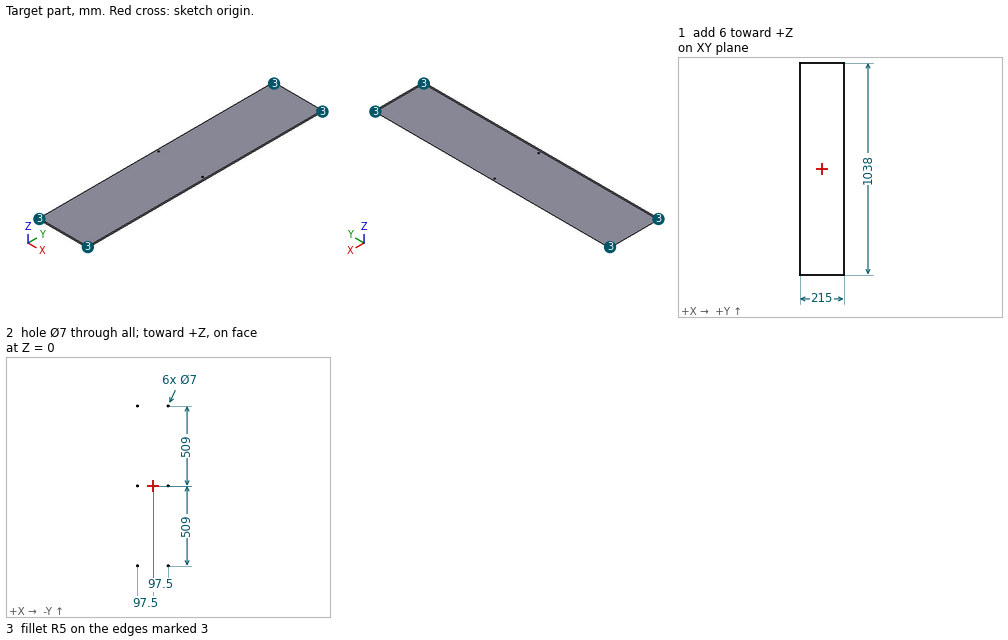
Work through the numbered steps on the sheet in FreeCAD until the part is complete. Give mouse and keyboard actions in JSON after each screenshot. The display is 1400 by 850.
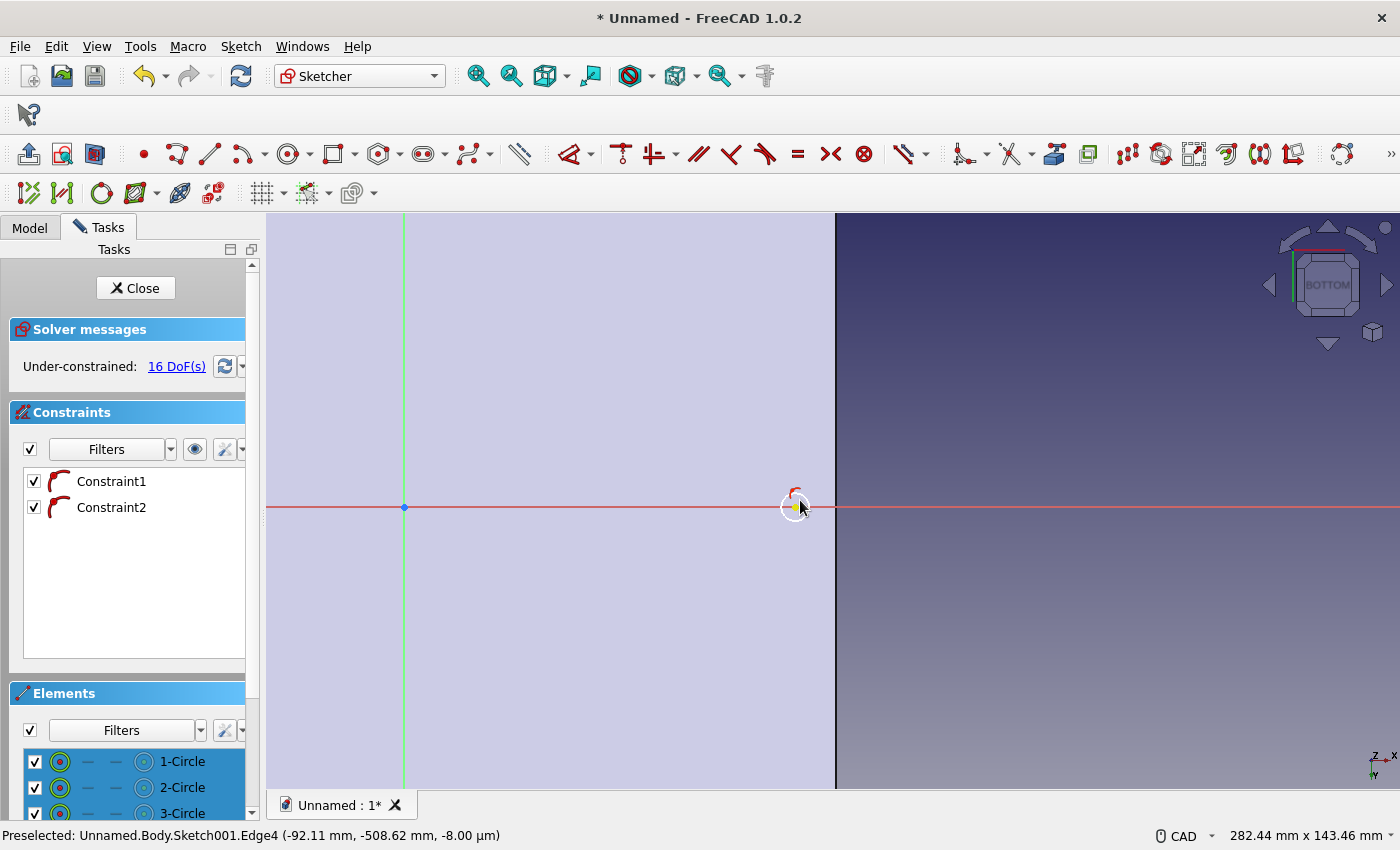
{"action": "left_click", "coordinate": [781, 507]}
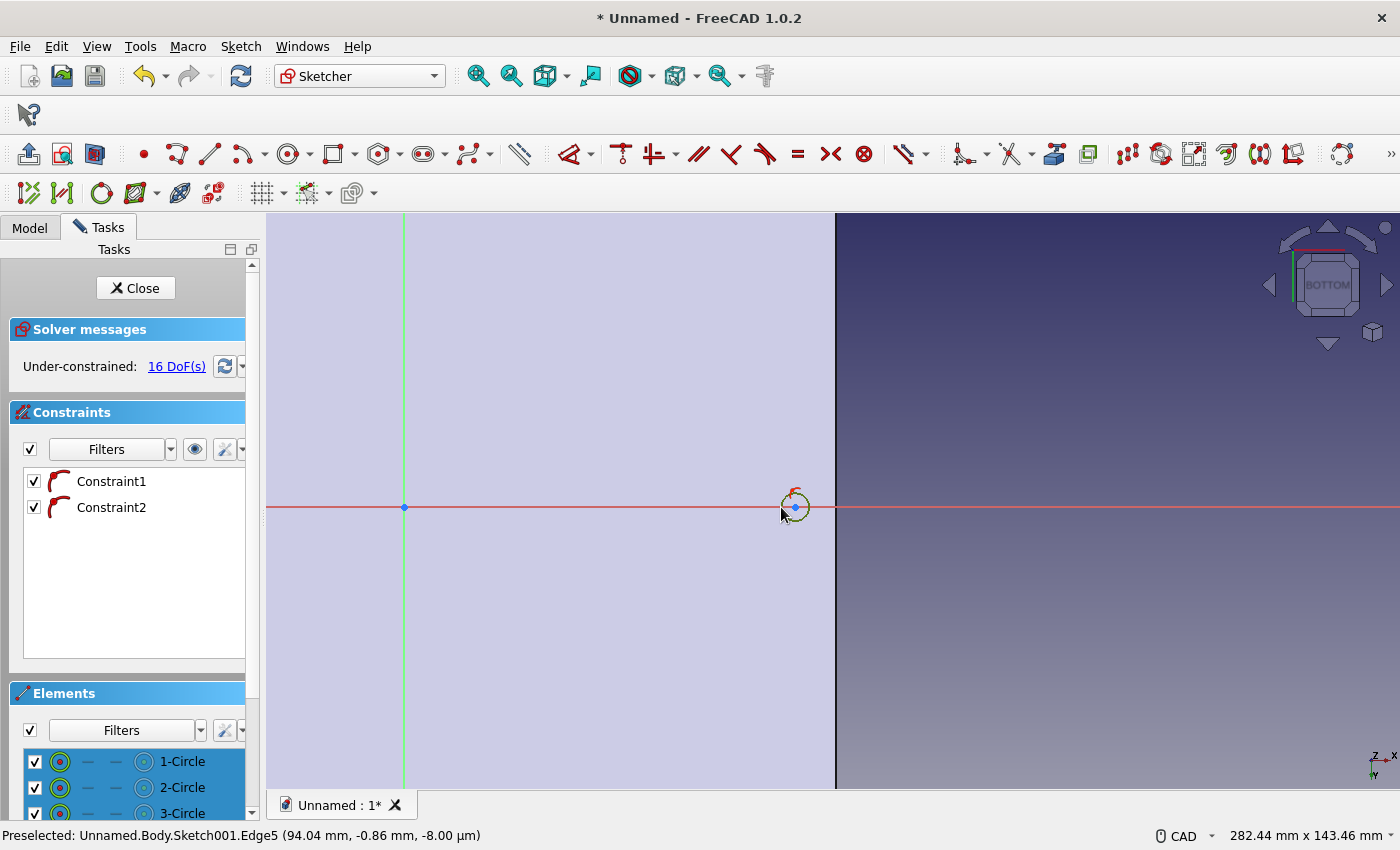
{"action": "scroll", "coordinate": [800, 500], "scroll_direction": "down", "scroll_amount": 12}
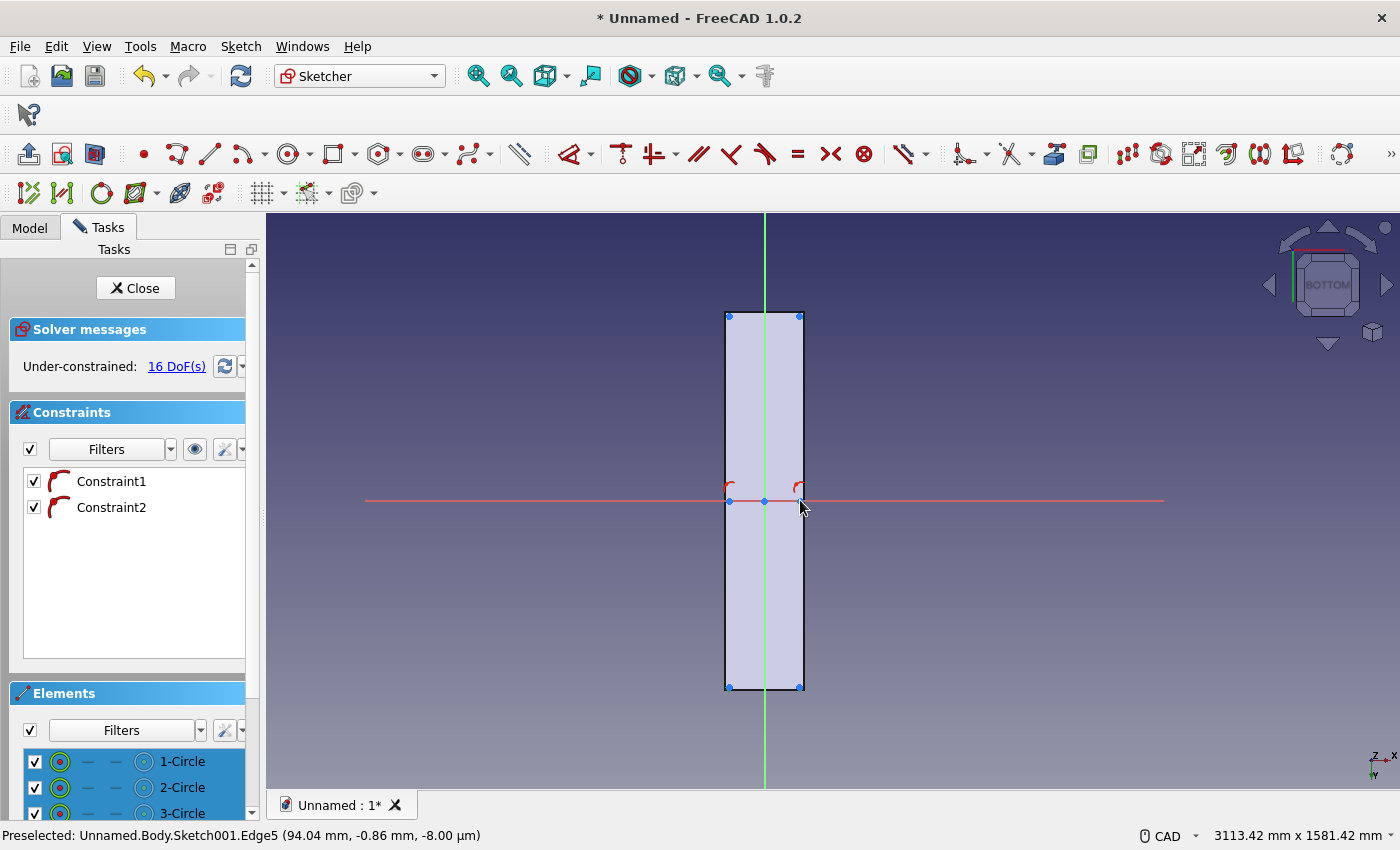
{"action": "scroll", "coordinate": [730, 500], "scroll_direction": "up", "scroll_amount": 14}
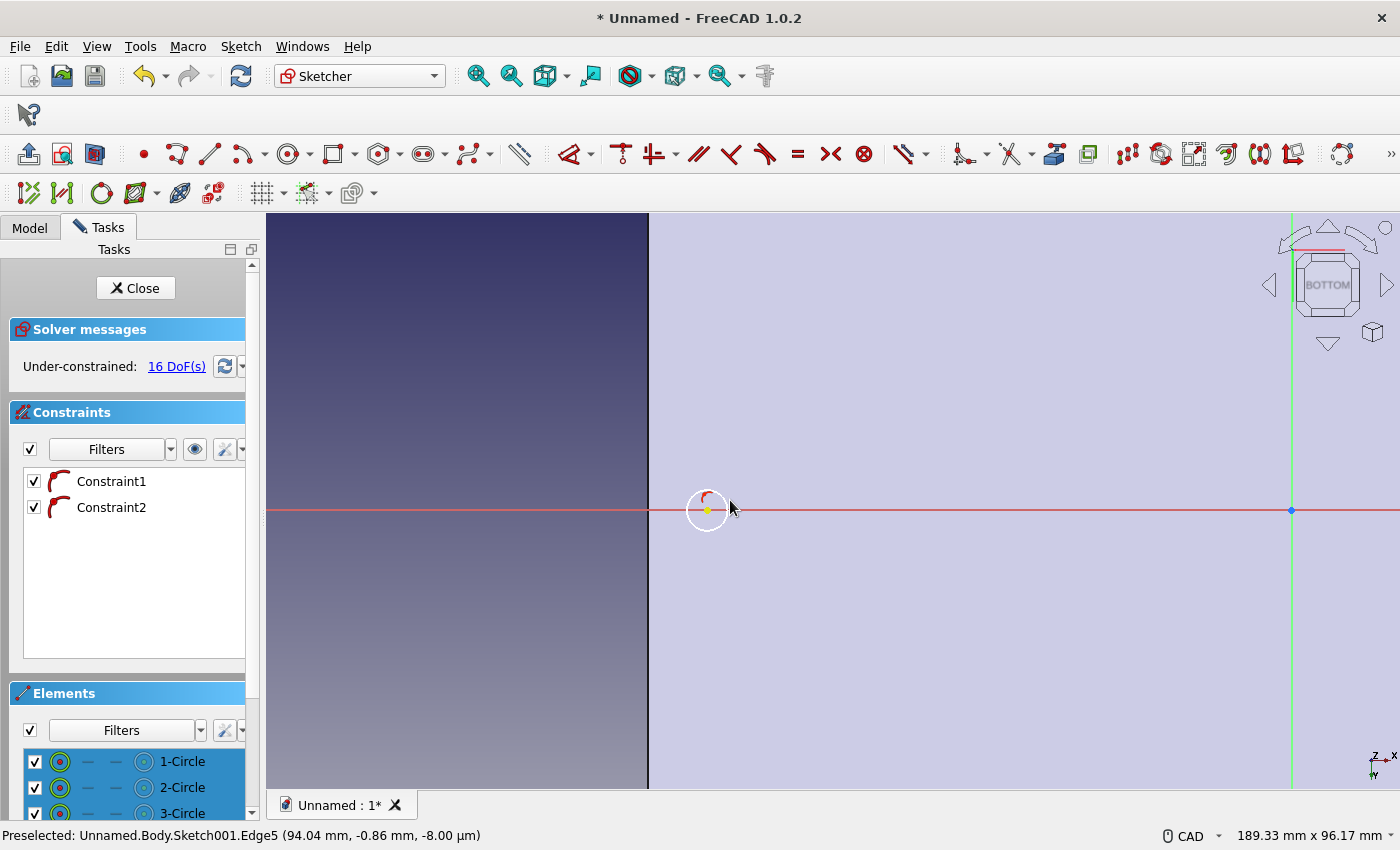
{"action": "left_click", "coordinate": [722, 496]}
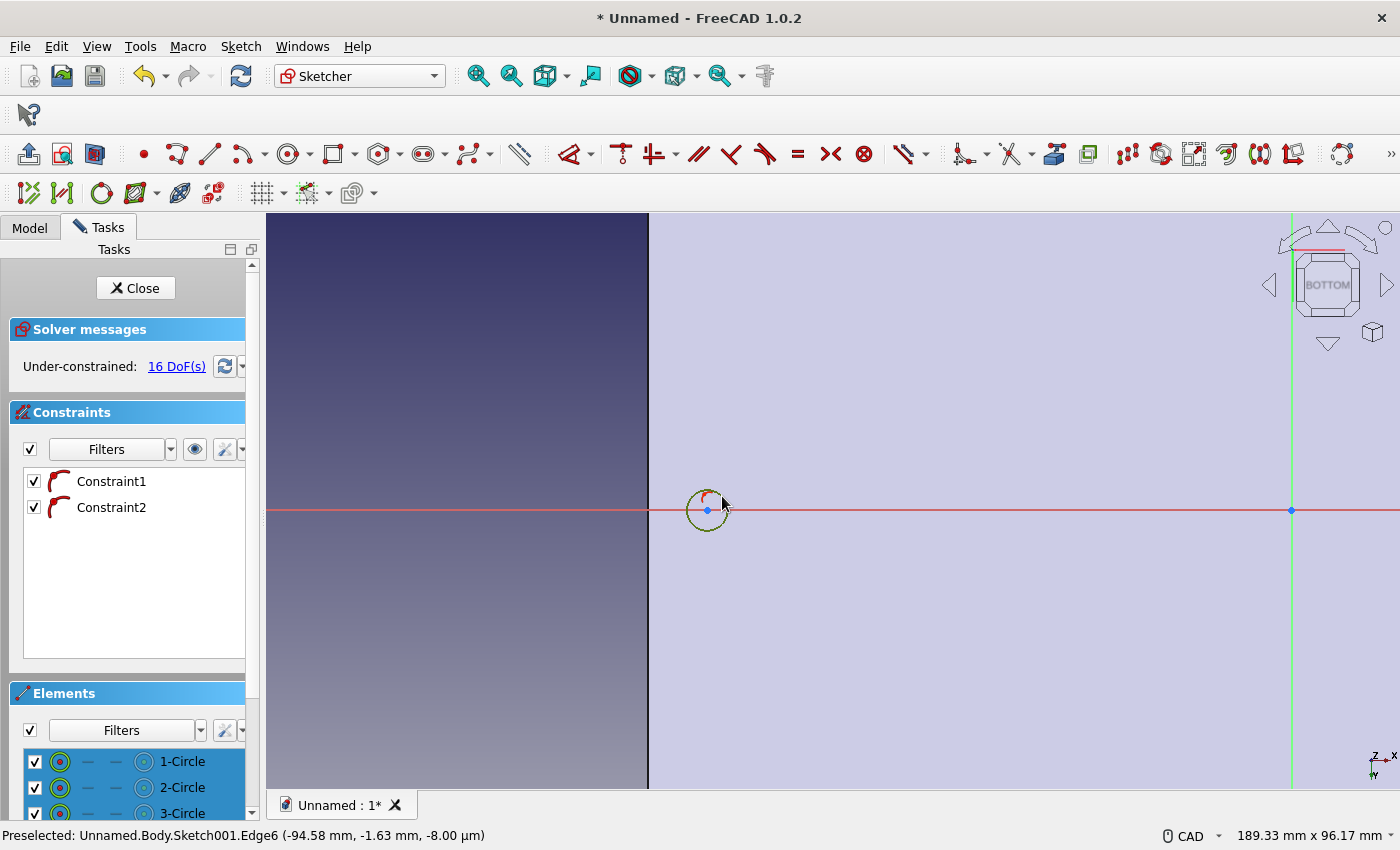
{"action": "left_click", "coordinate": [798, 154]}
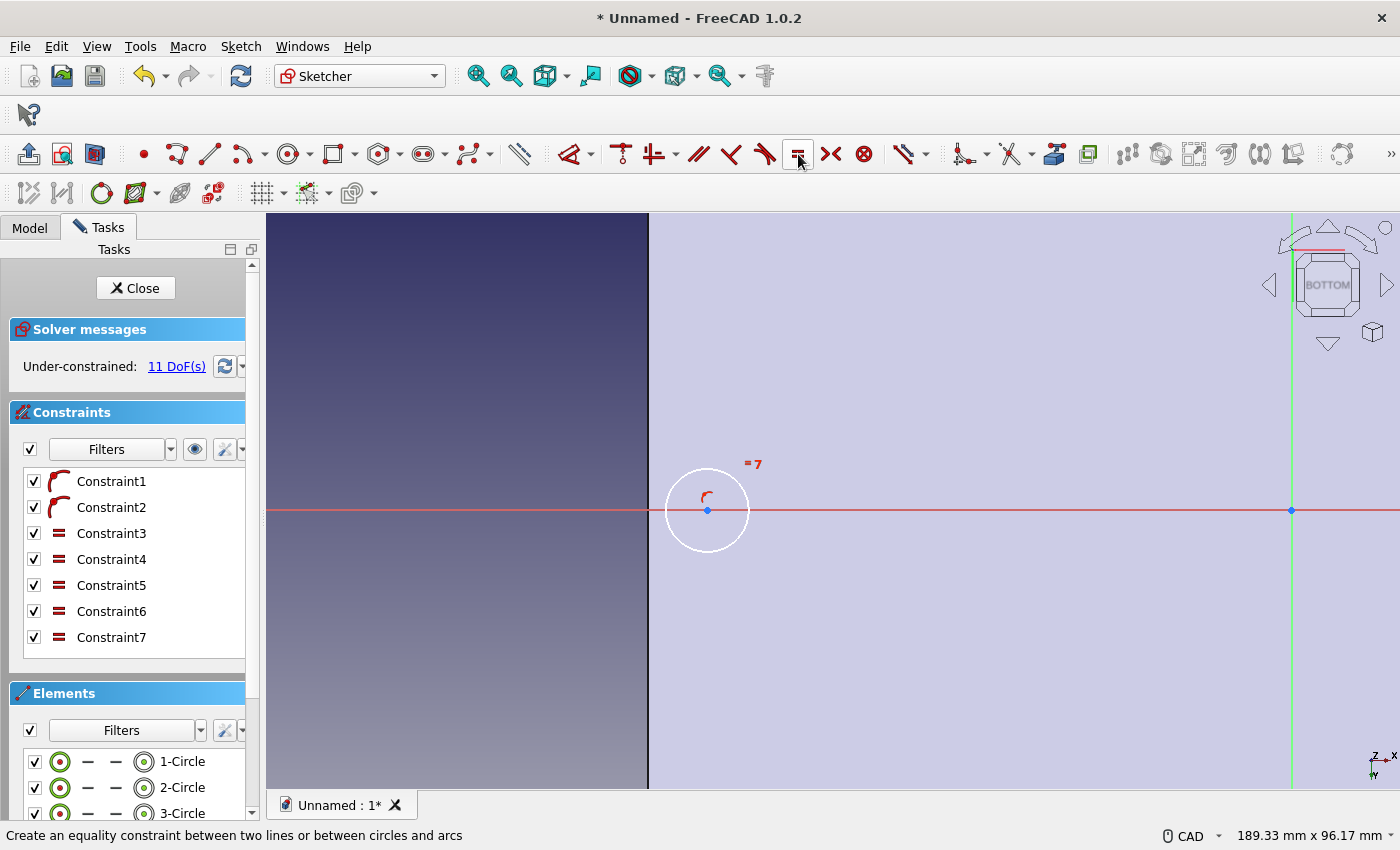
{"action": "scroll", "coordinate": [730, 500], "scroll_direction": "down", "scroll_amount": 14}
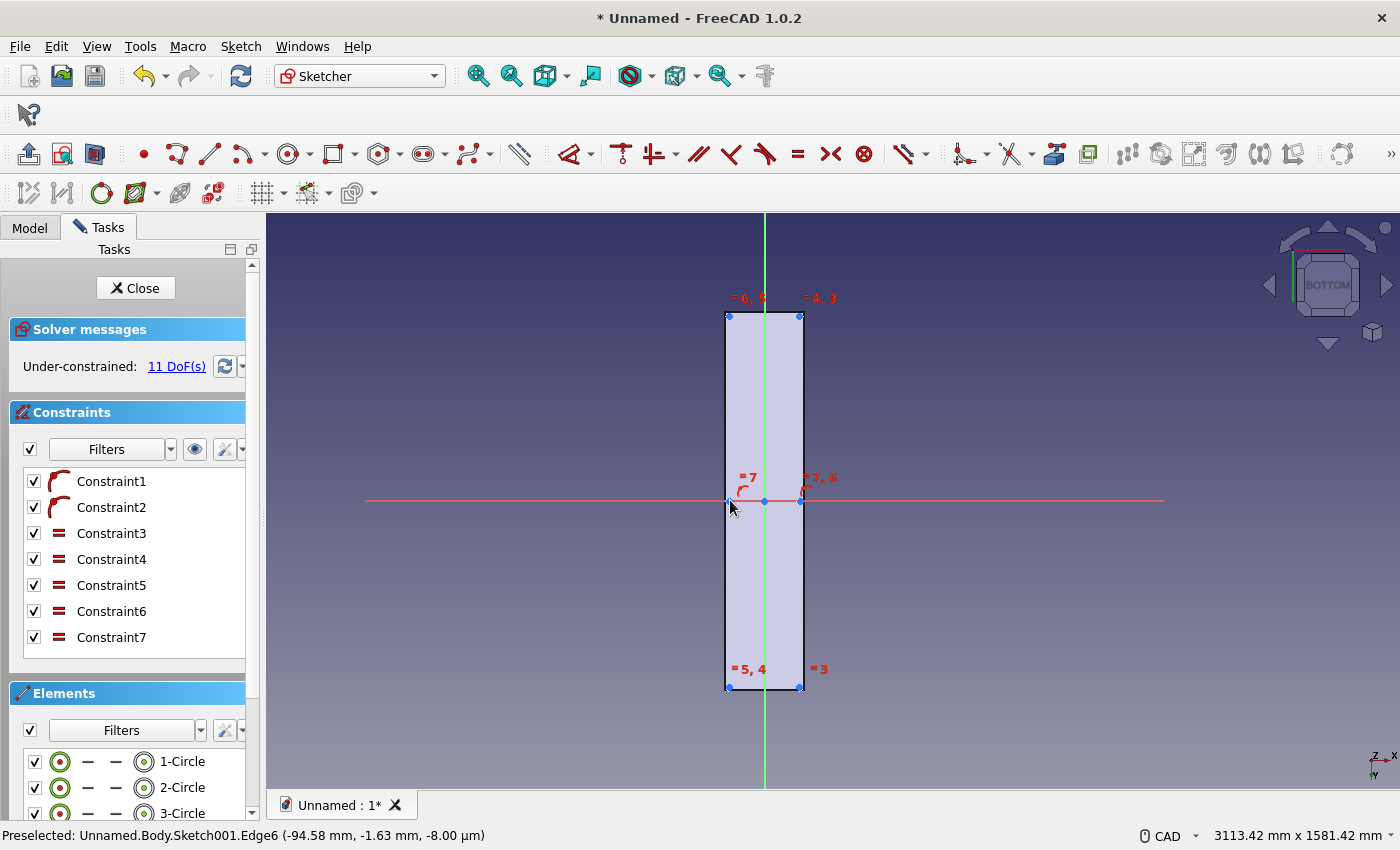
{"action": "left_click", "coordinate": [800, 688]}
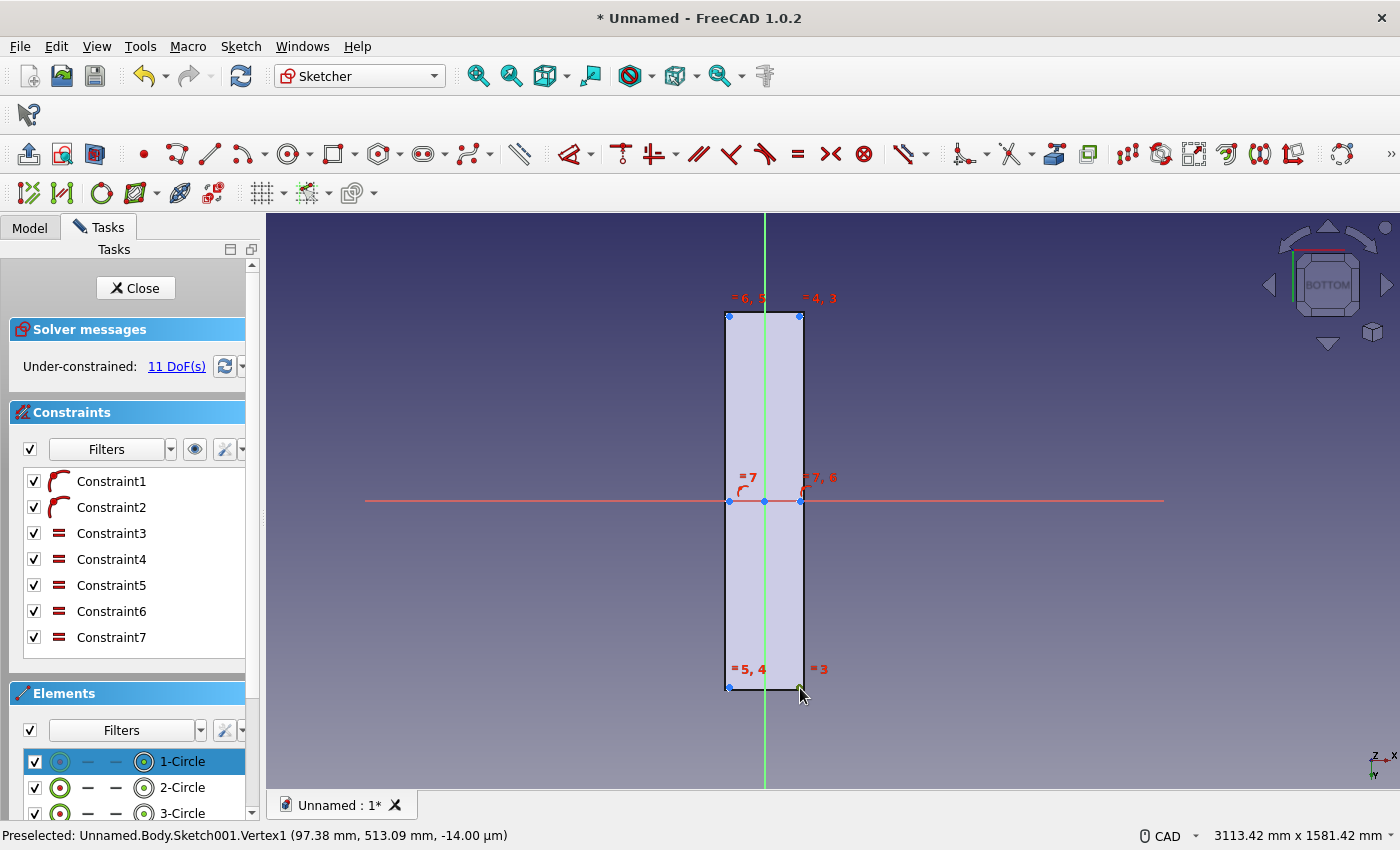
{"action": "left_click", "coordinate": [800, 317]}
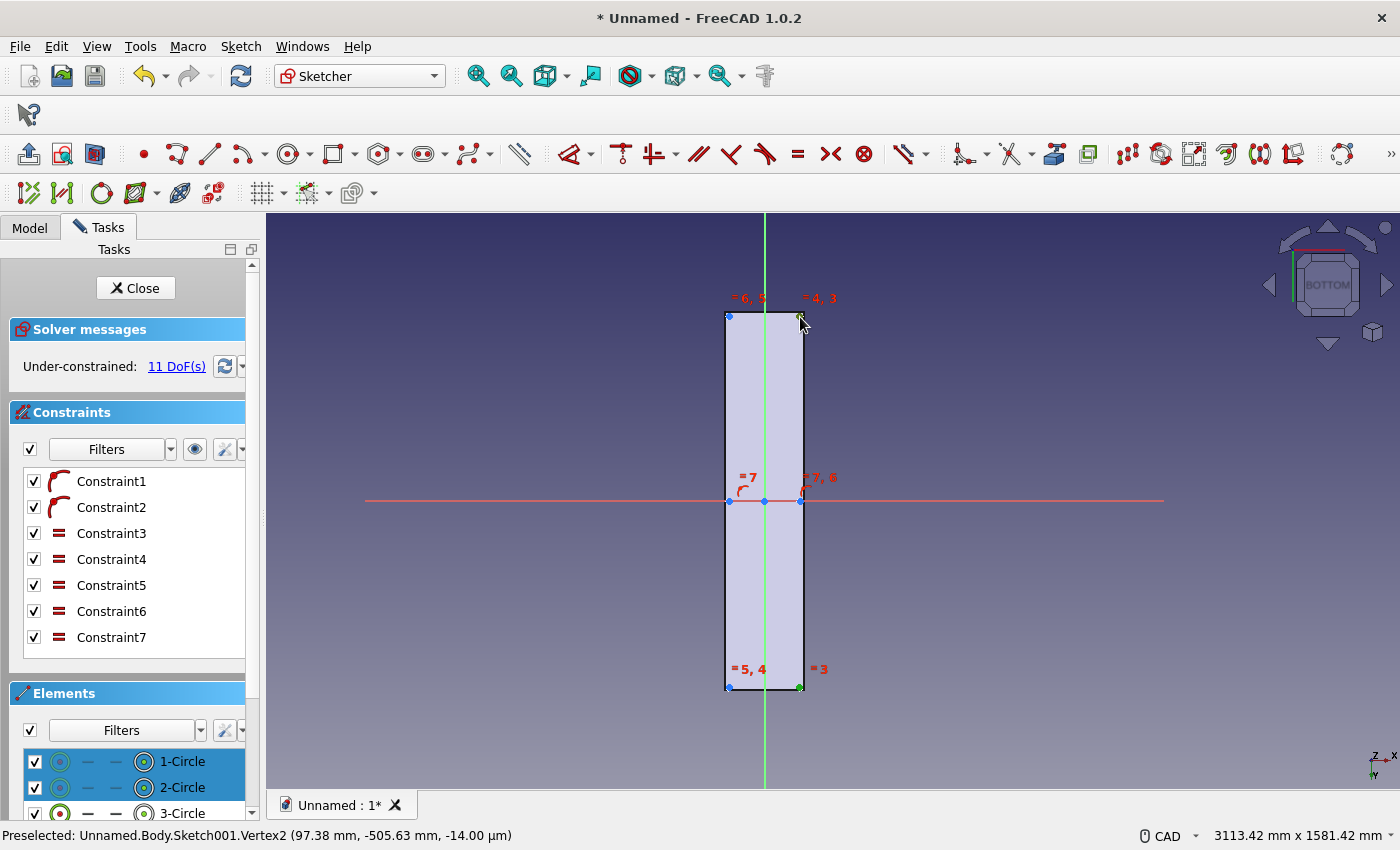
{"action": "key", "text": "v"}